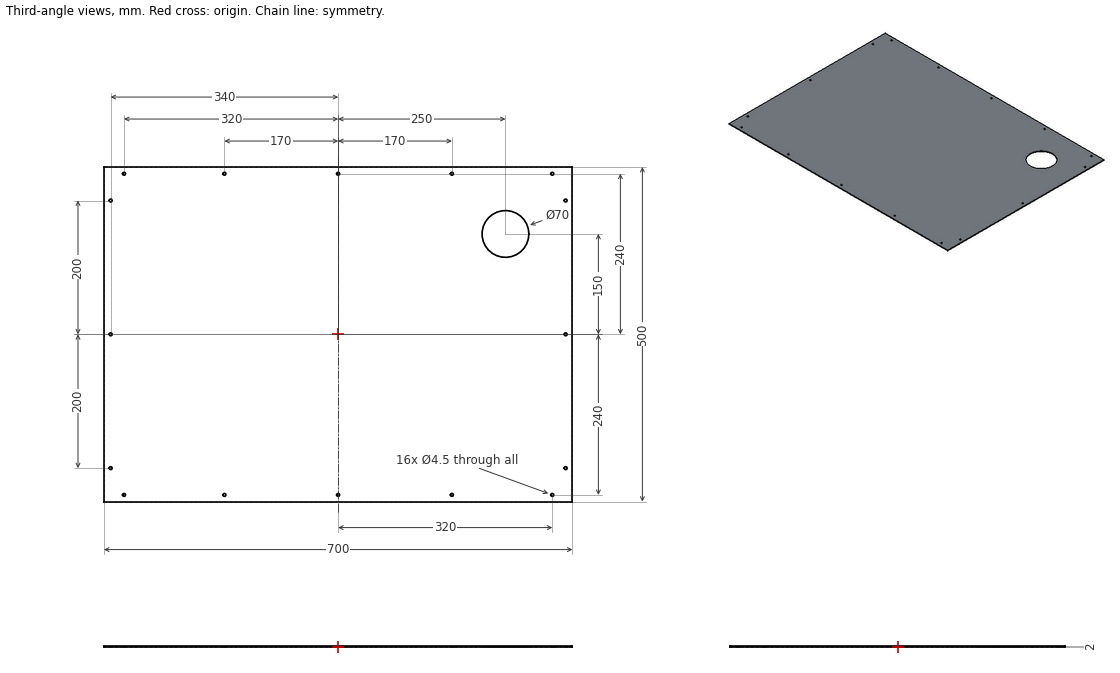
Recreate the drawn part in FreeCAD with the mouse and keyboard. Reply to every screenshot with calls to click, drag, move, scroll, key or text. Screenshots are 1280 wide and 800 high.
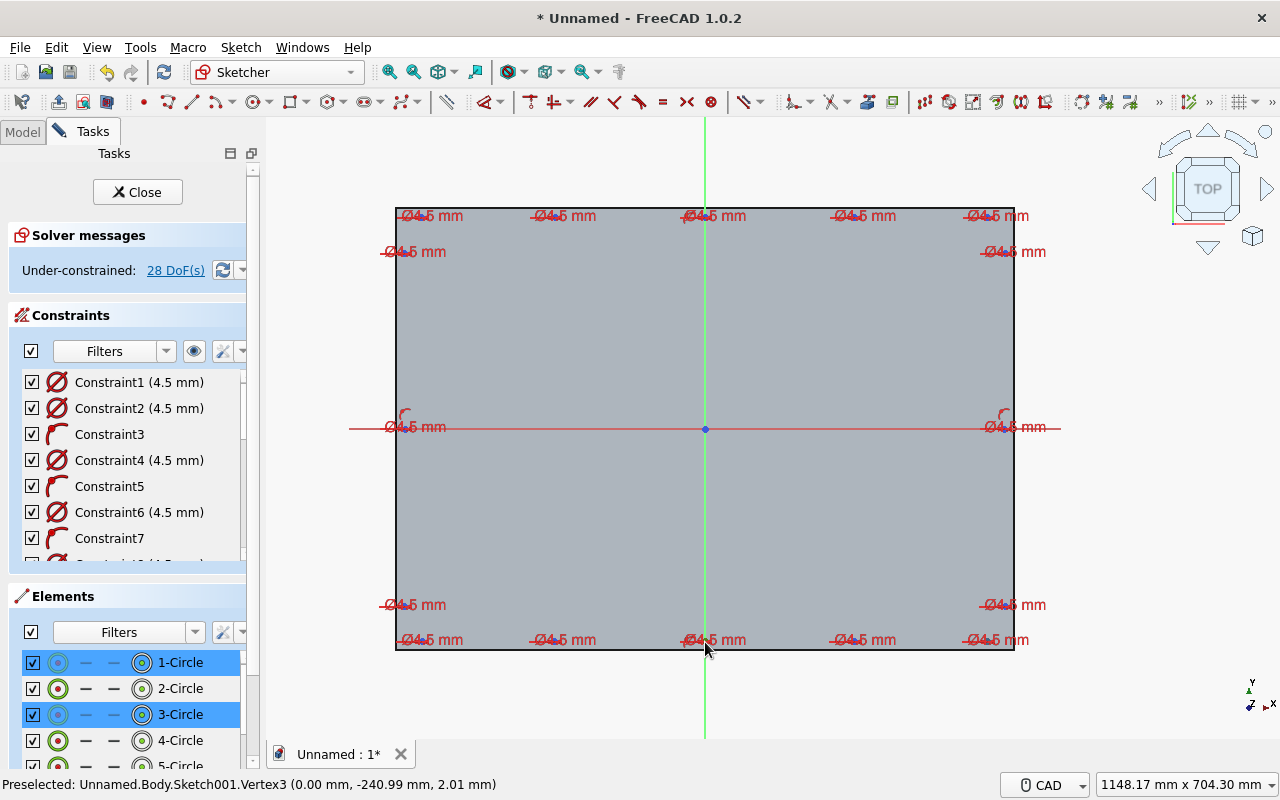
key(h)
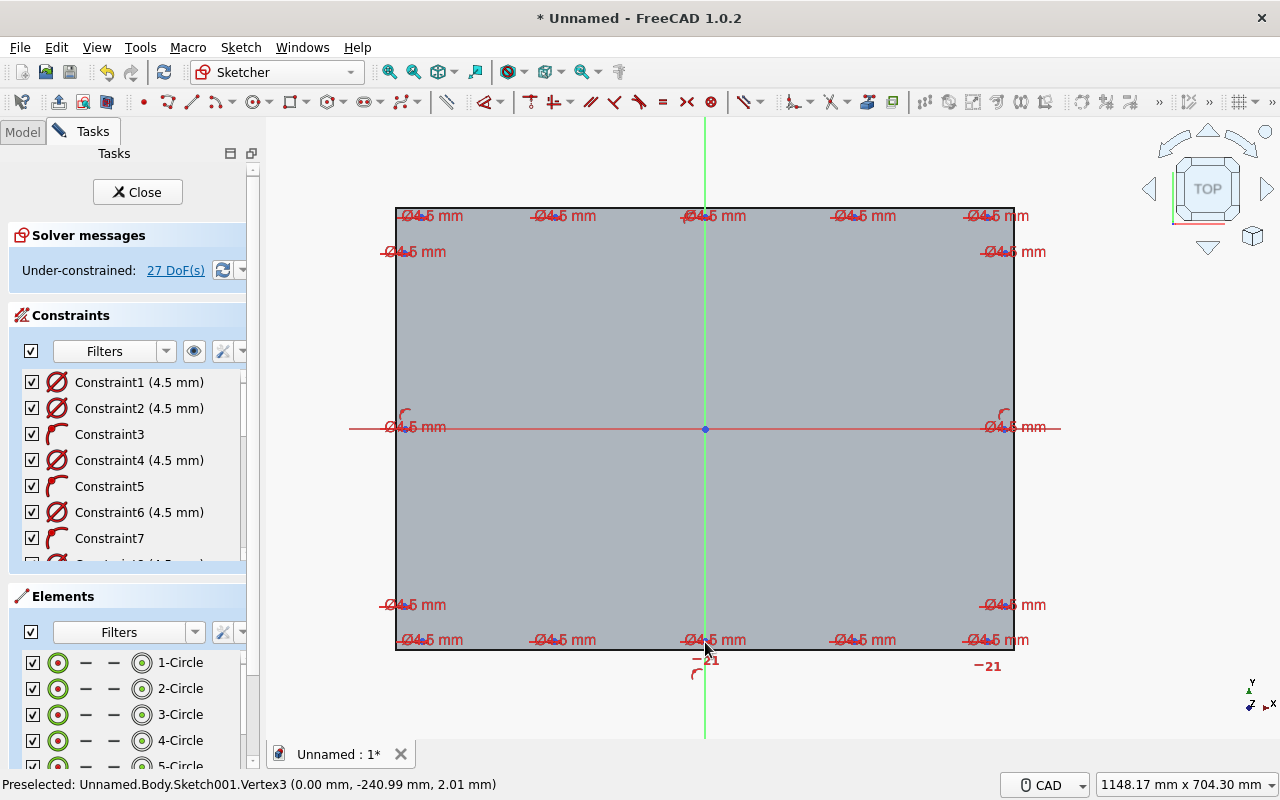
click(705, 218)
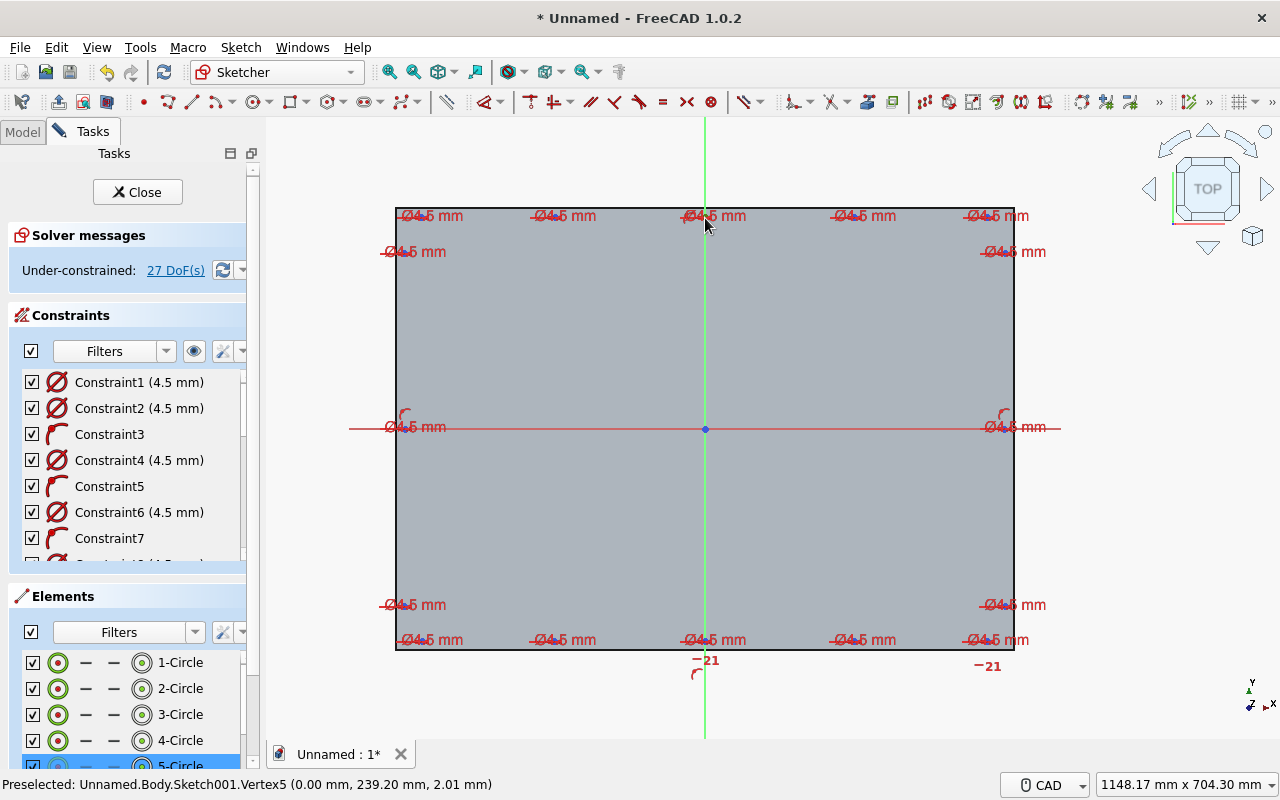
click(555, 218)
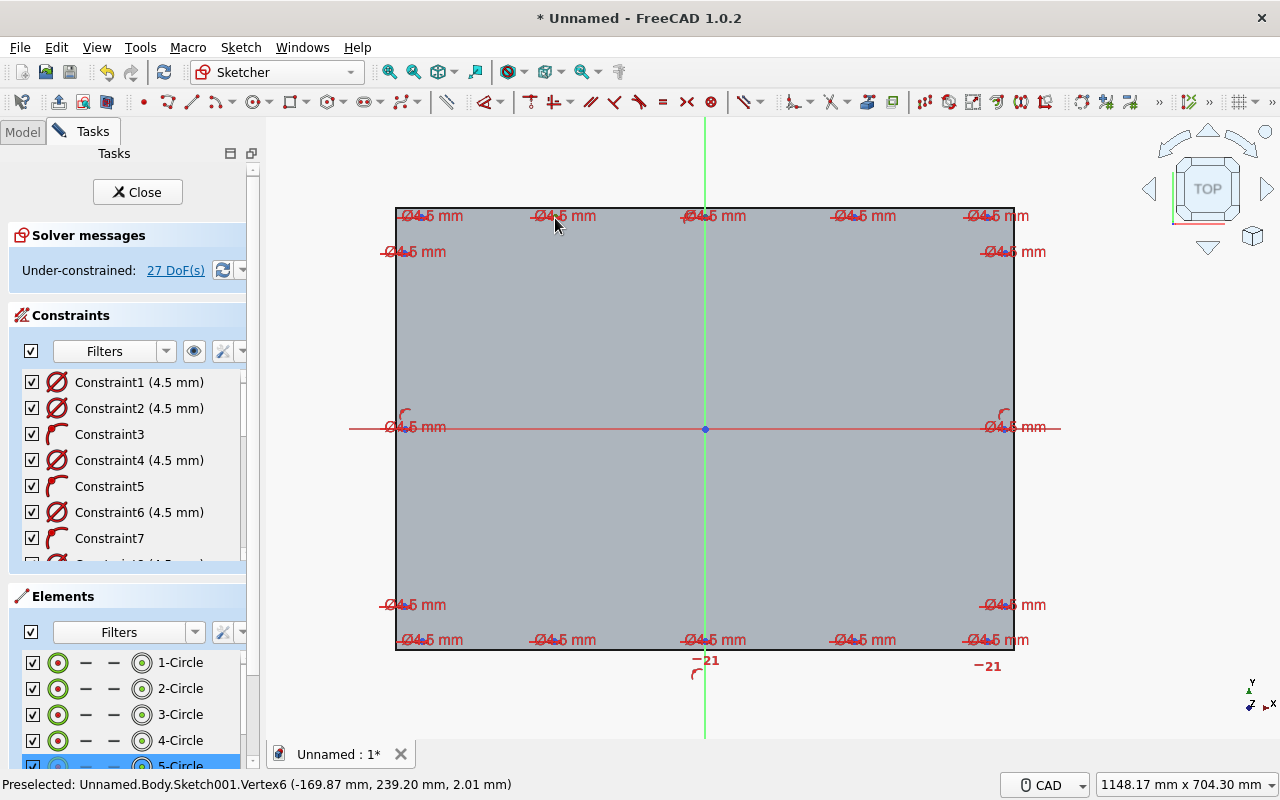
click(572, 102)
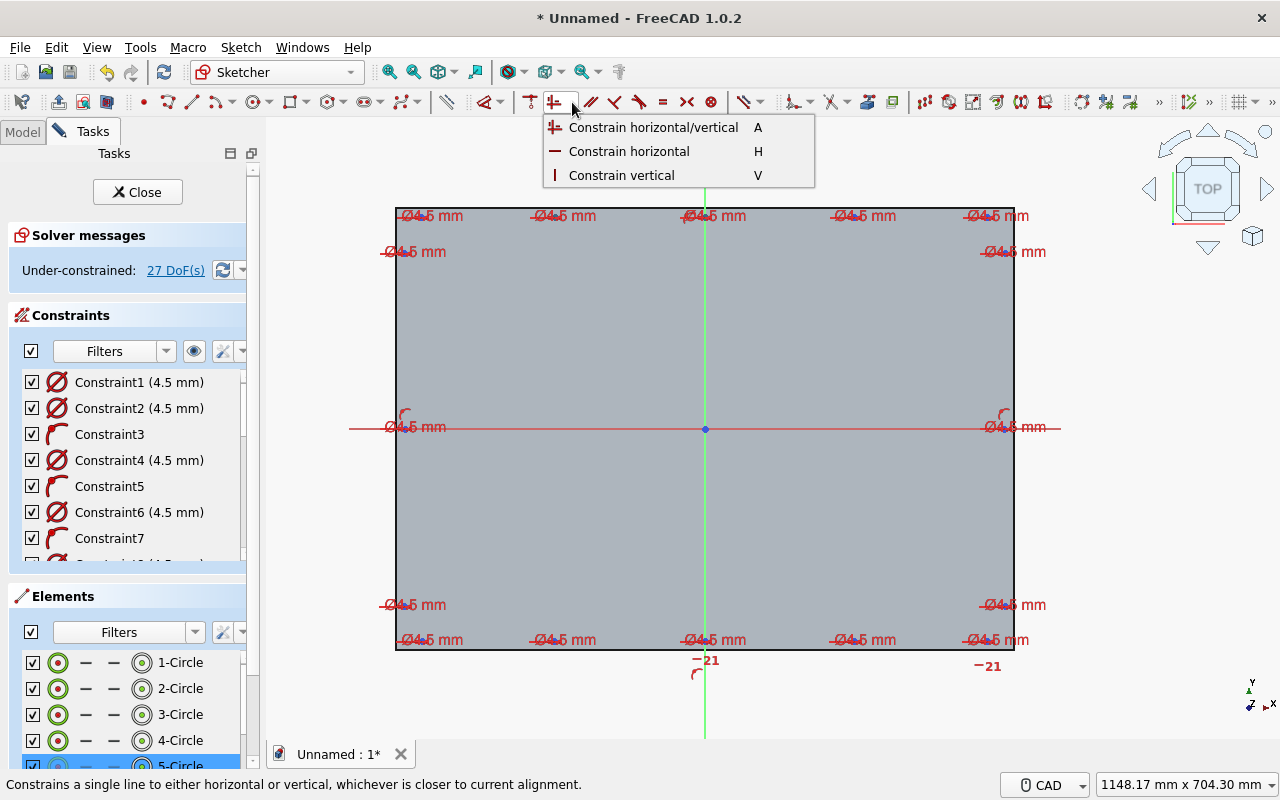
click(679, 151)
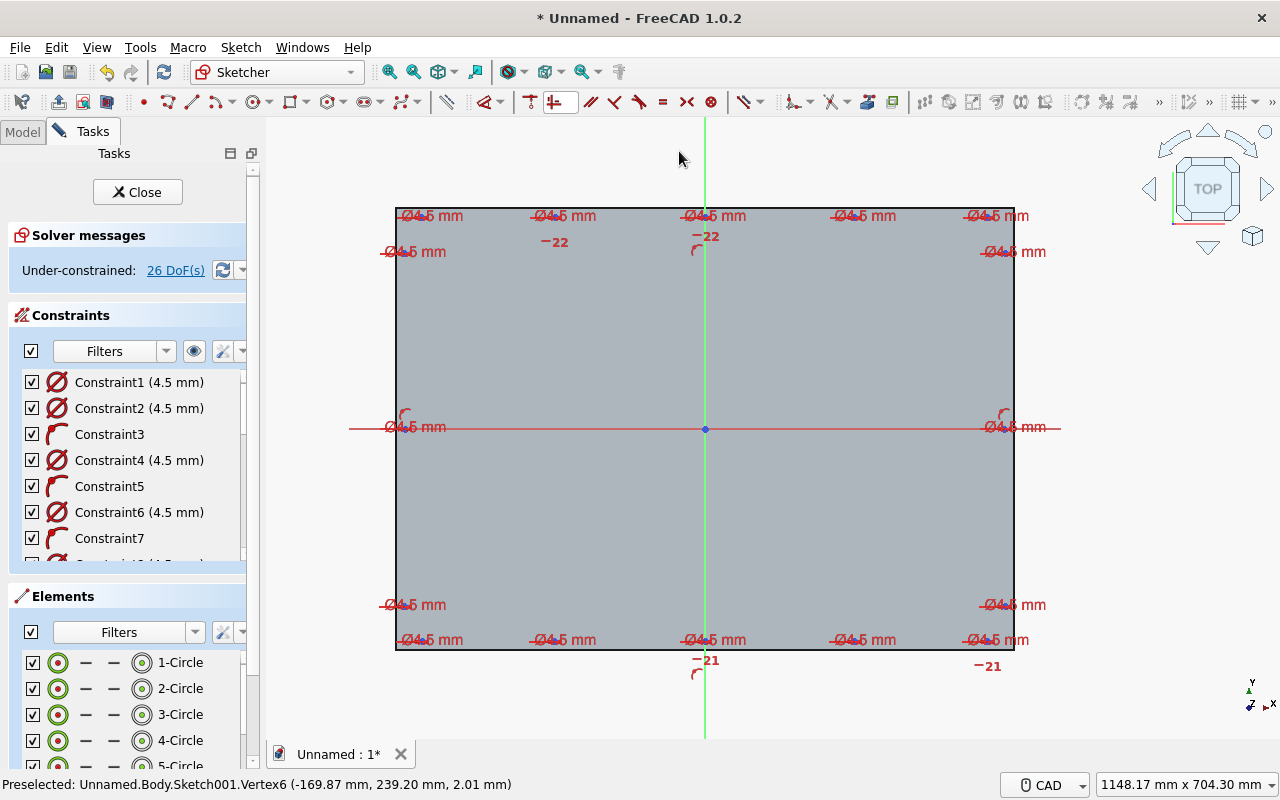
click(705, 218)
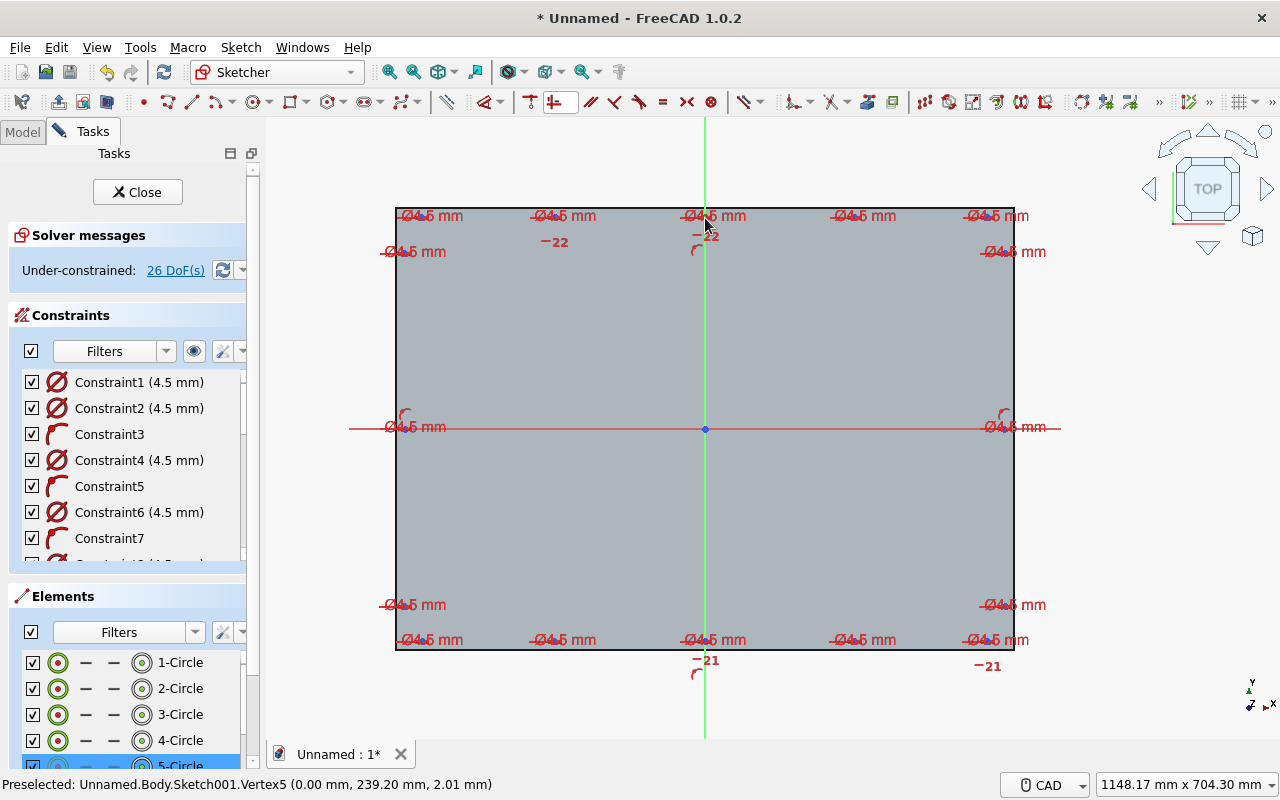
click(855, 218)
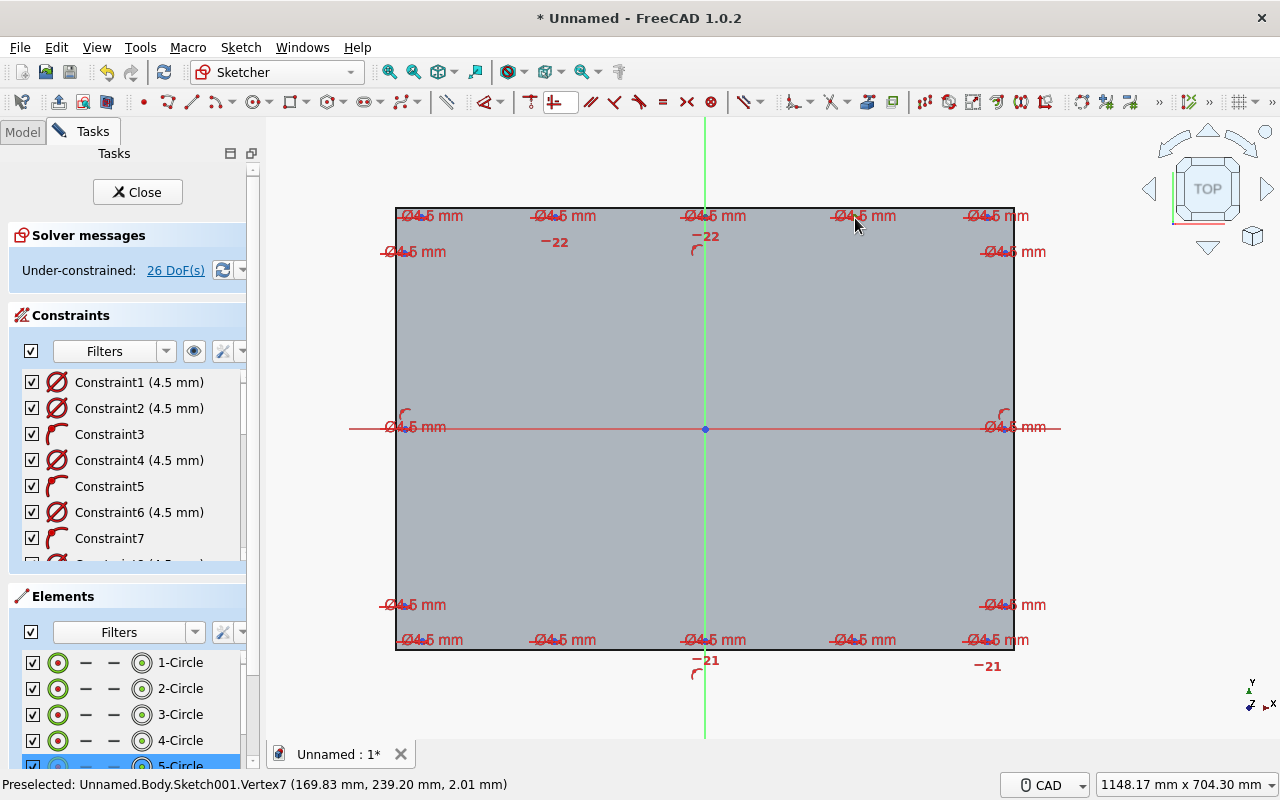
key(h)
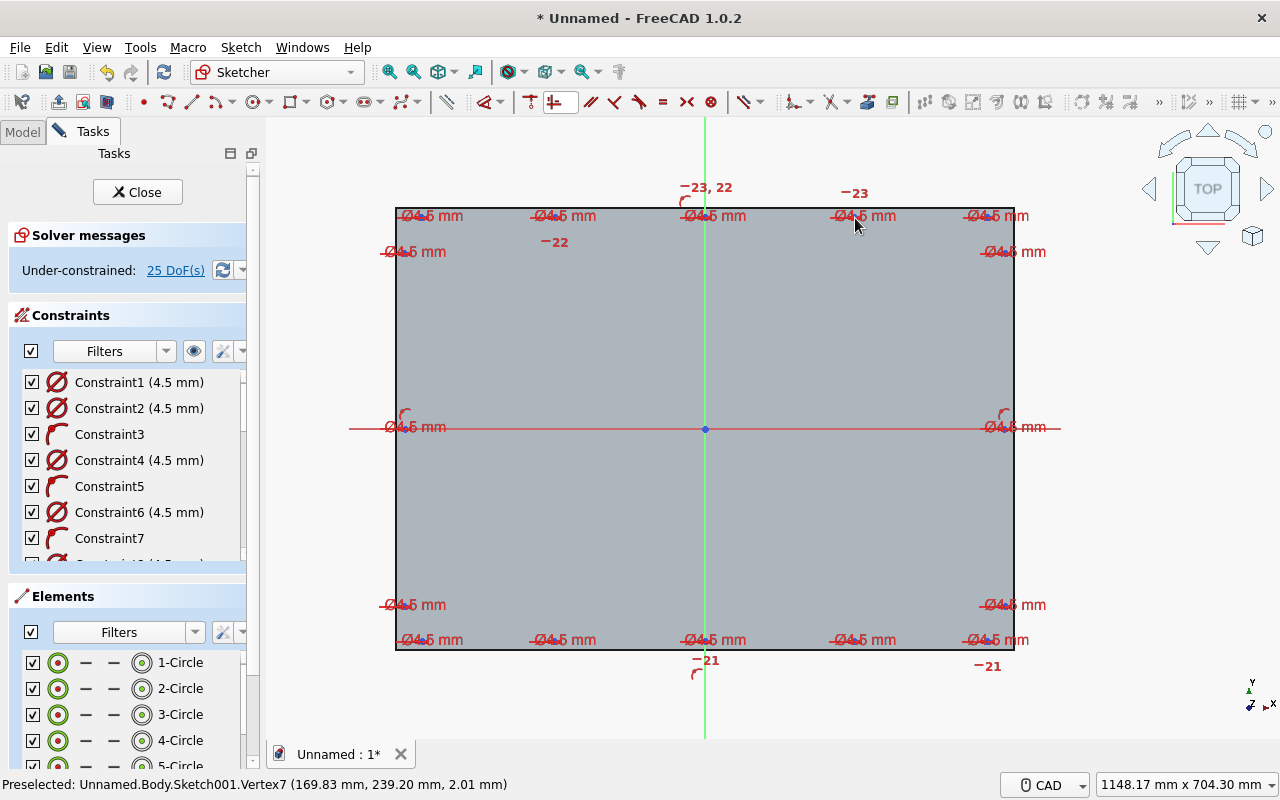
click(555, 218)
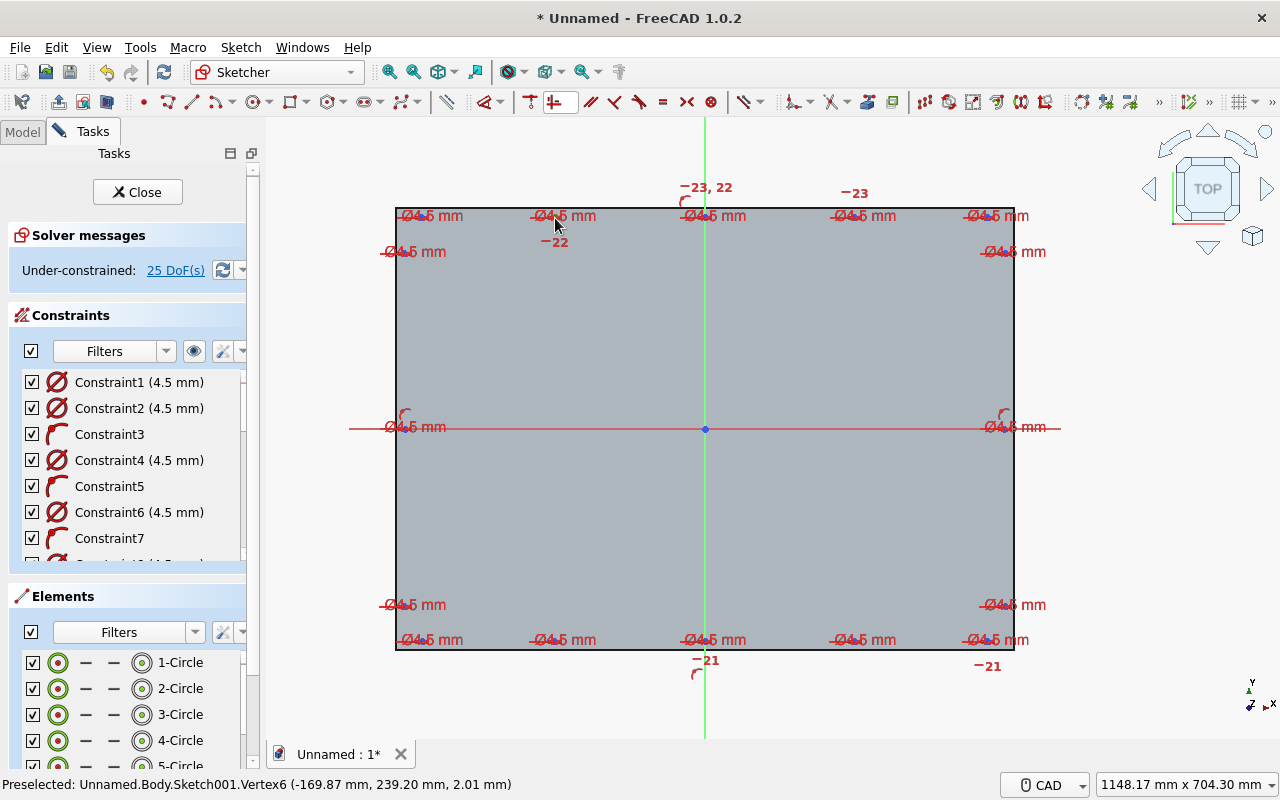
click(555, 642)